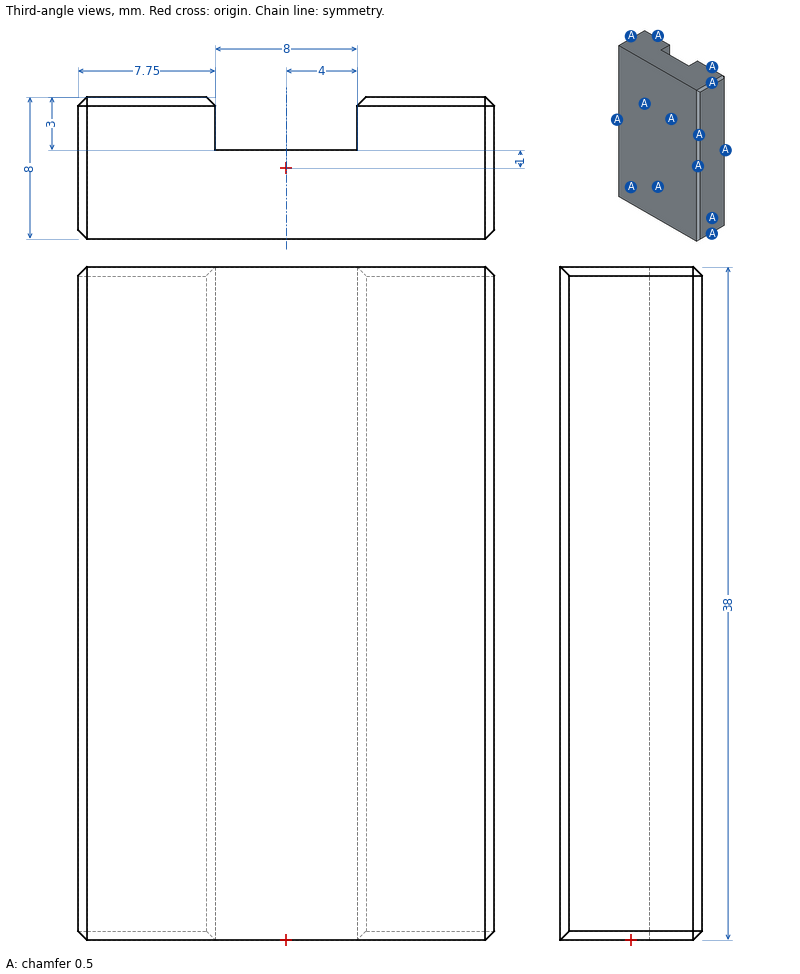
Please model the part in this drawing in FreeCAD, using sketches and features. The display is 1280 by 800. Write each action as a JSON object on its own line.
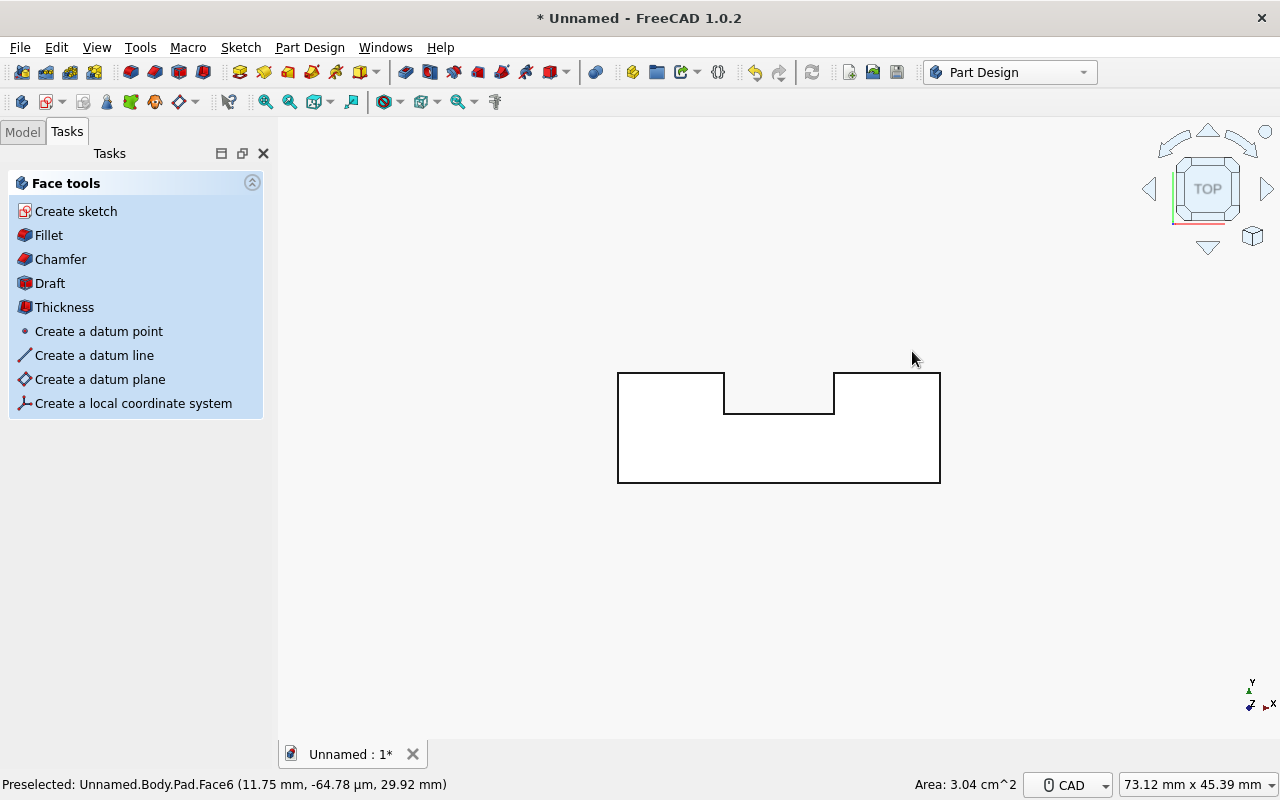
{"action": "key", "text": "1"}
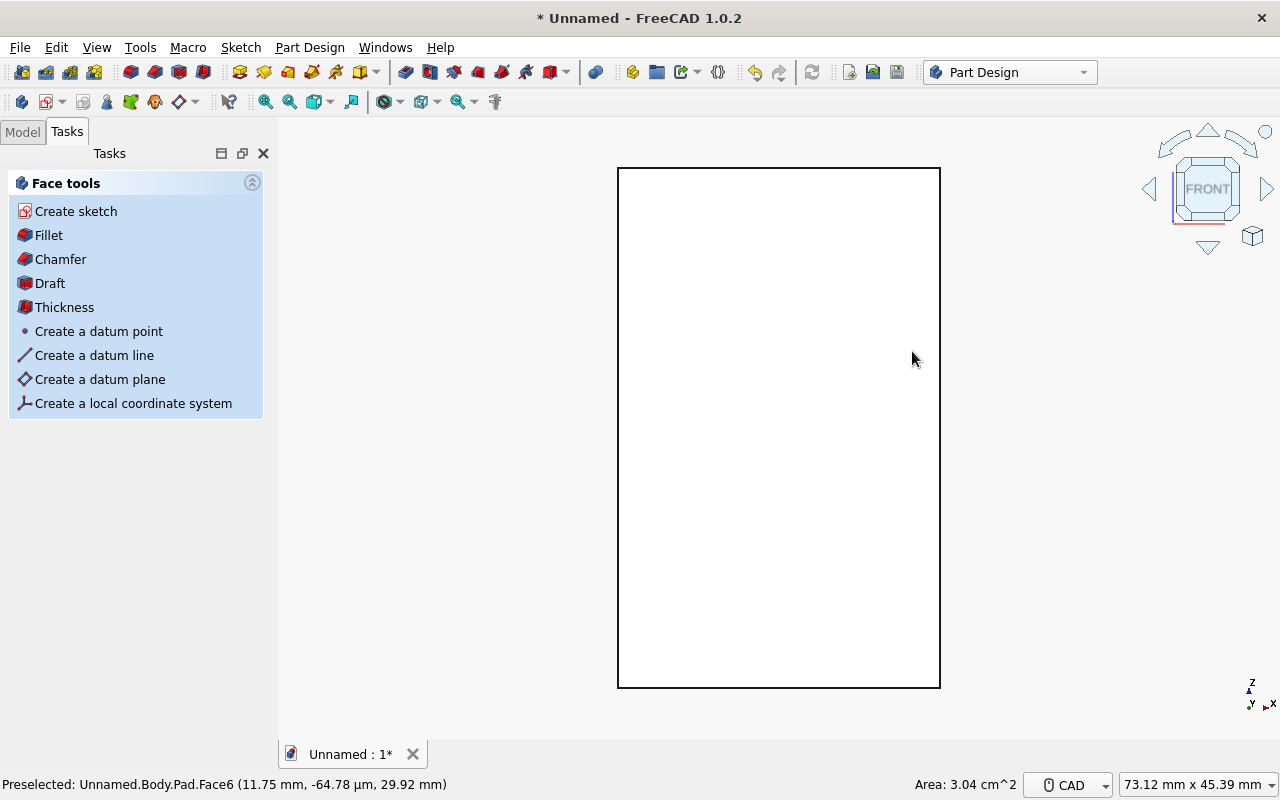
{"action": "key", "text": "3"}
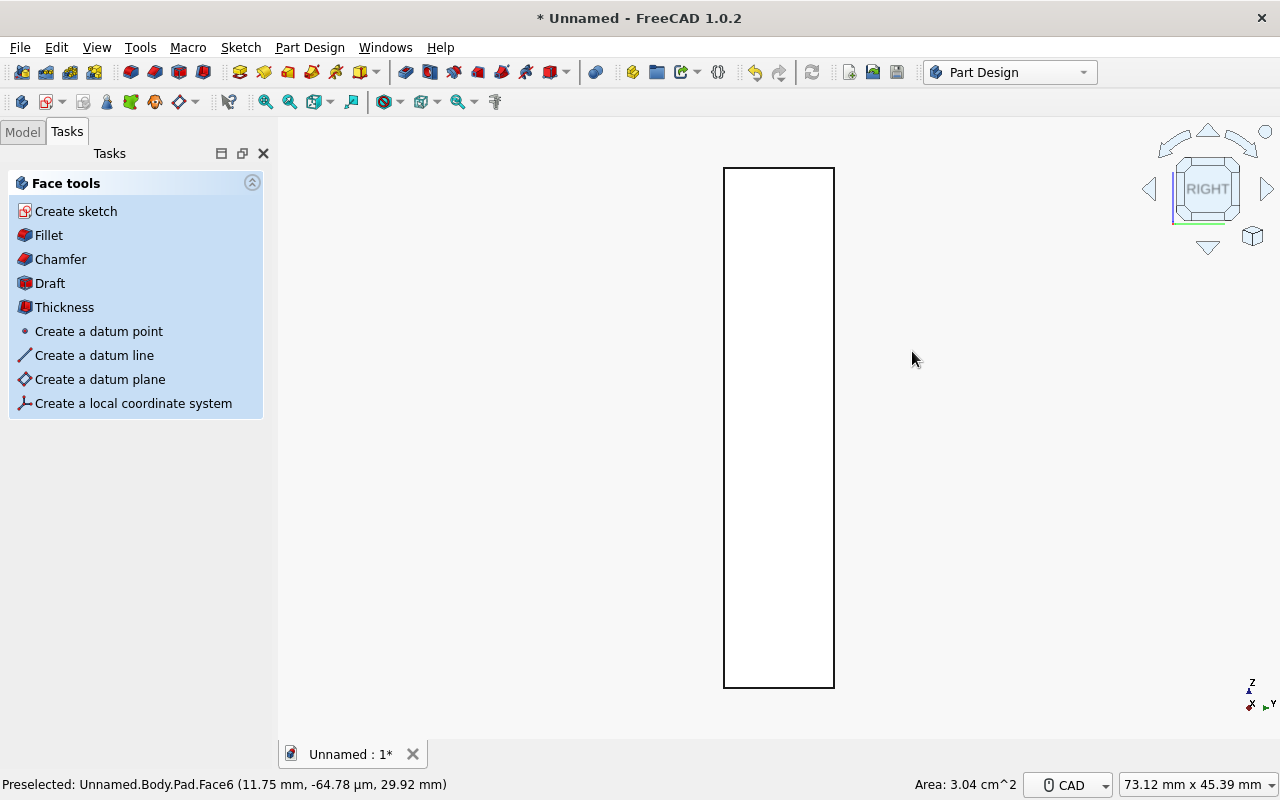
{"action": "key", "text": "5"}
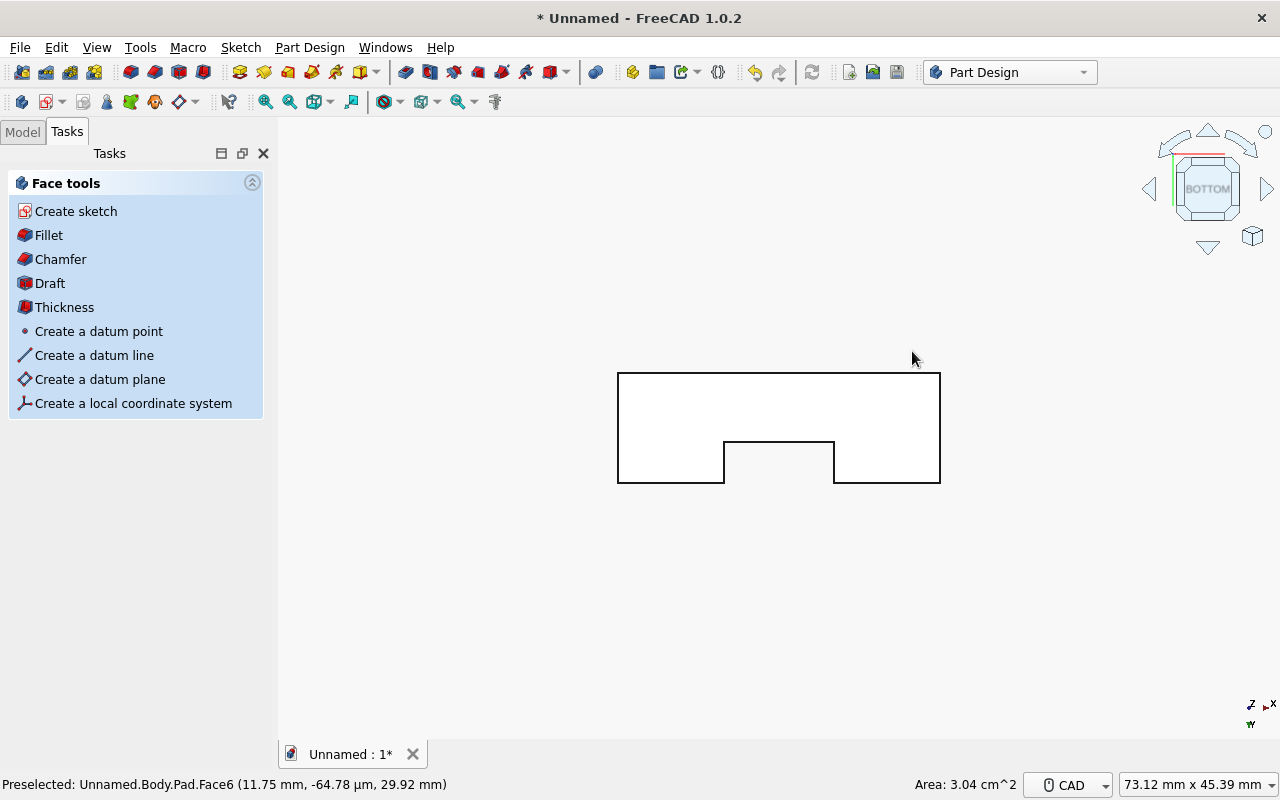
{"action": "left_click", "coordinate": [266, 102]}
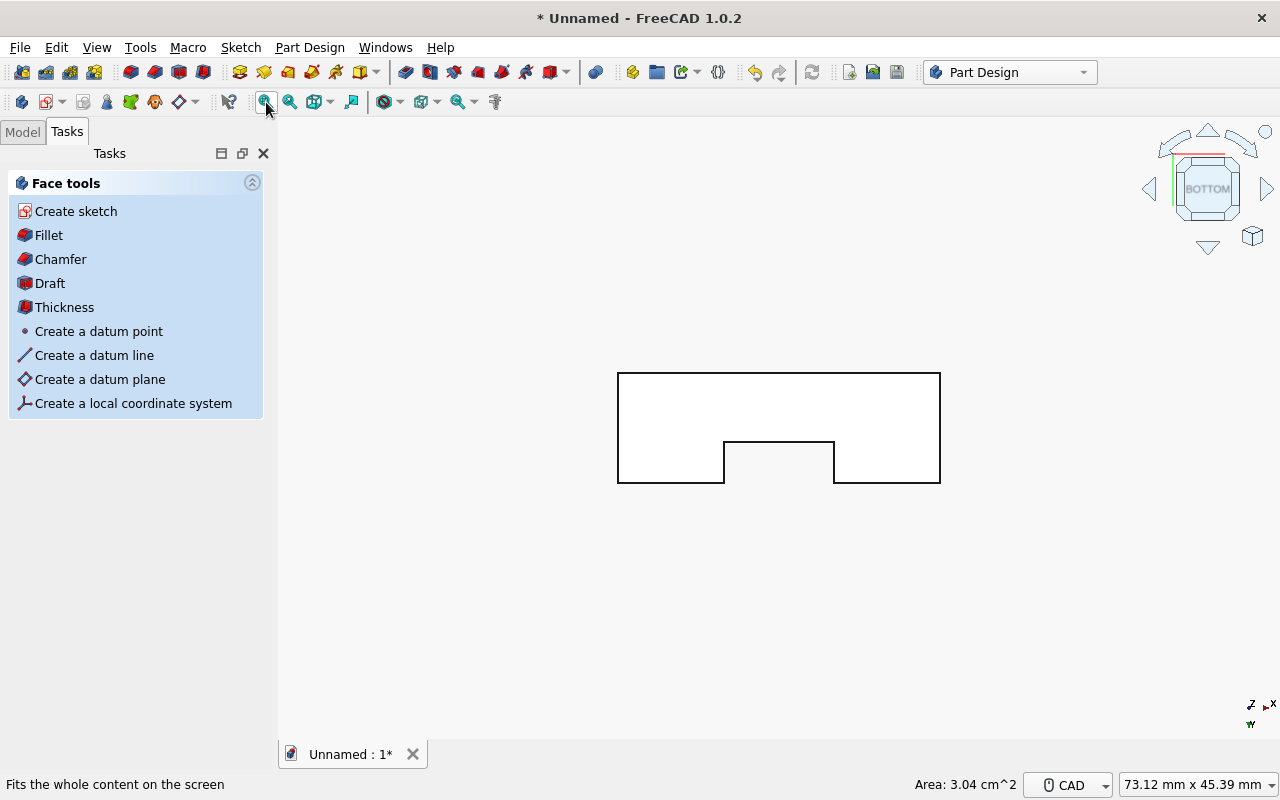
{"action": "key", "text": "4"}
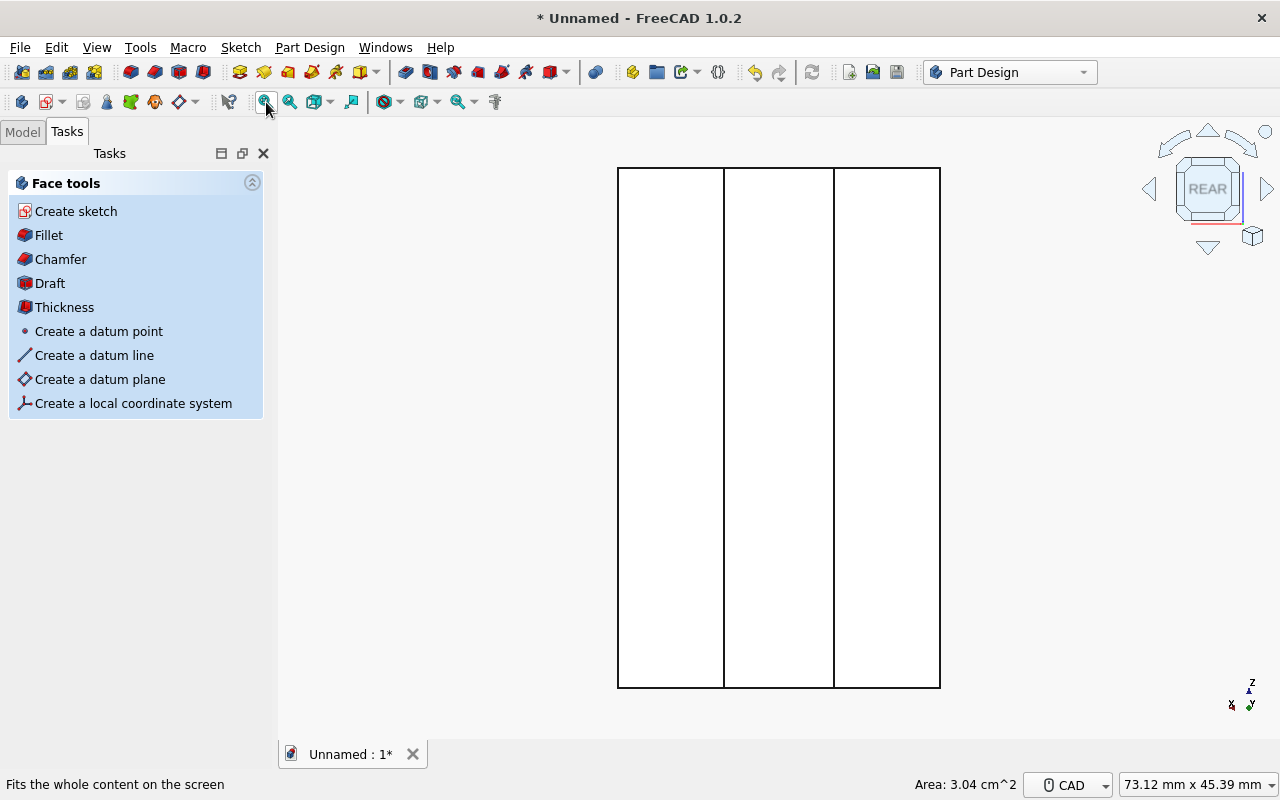
{"action": "left_click", "coordinate": [887, 278], "text": "ctrl"}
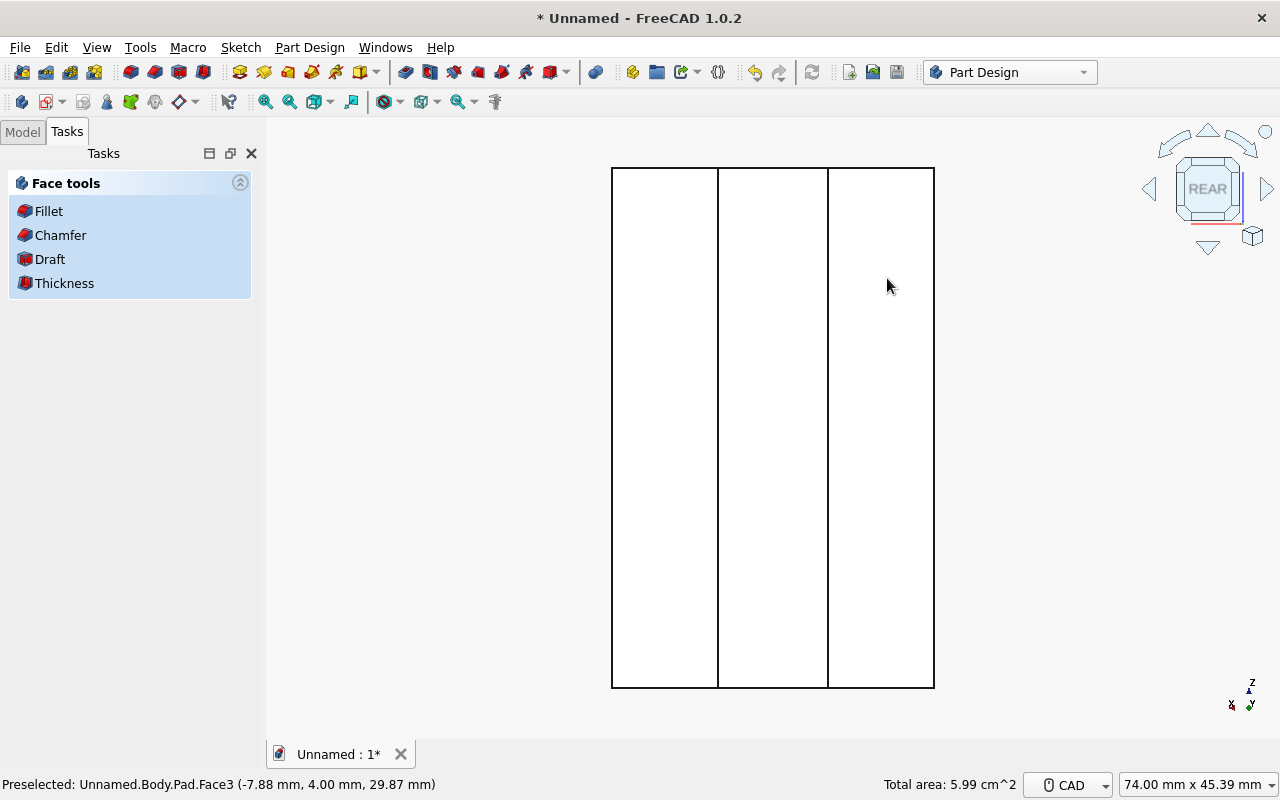
{"action": "left_click", "coordinate": [665, 278], "text": "ctrl"}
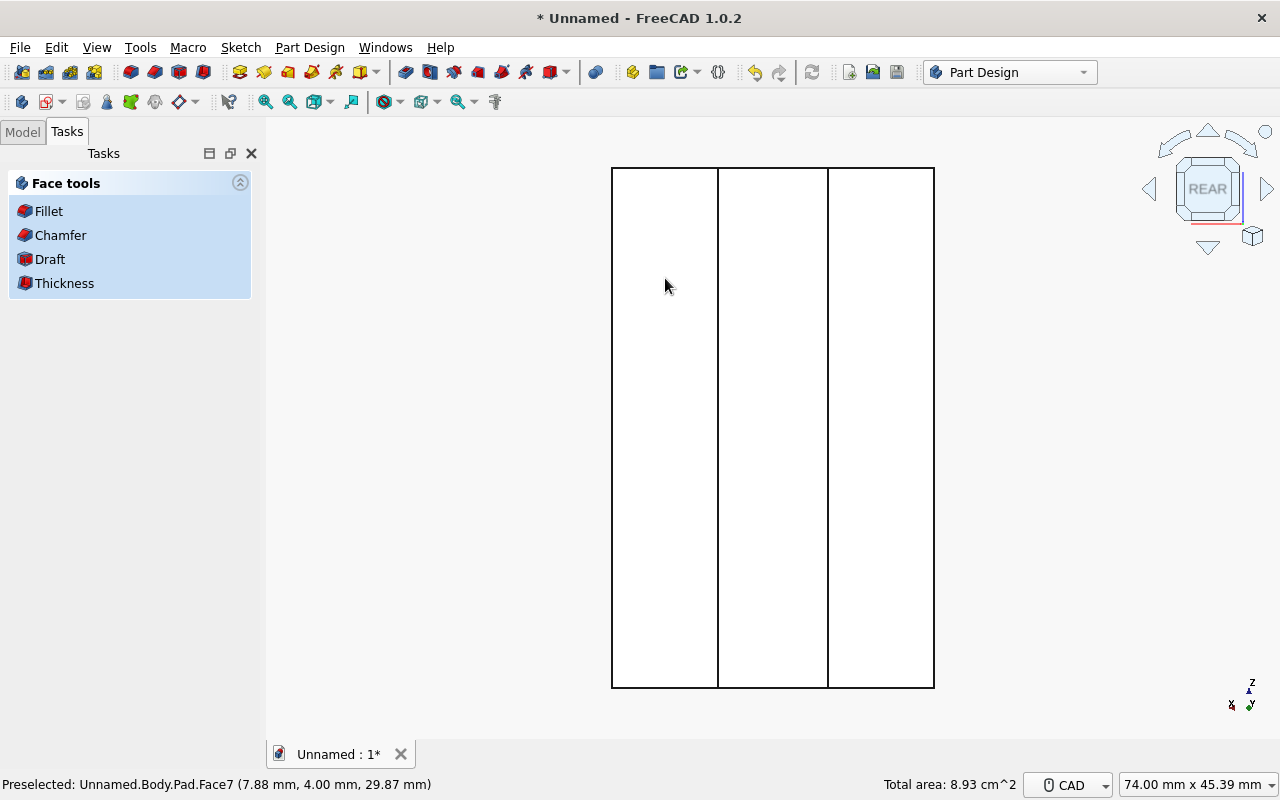
{"action": "key", "text": "6"}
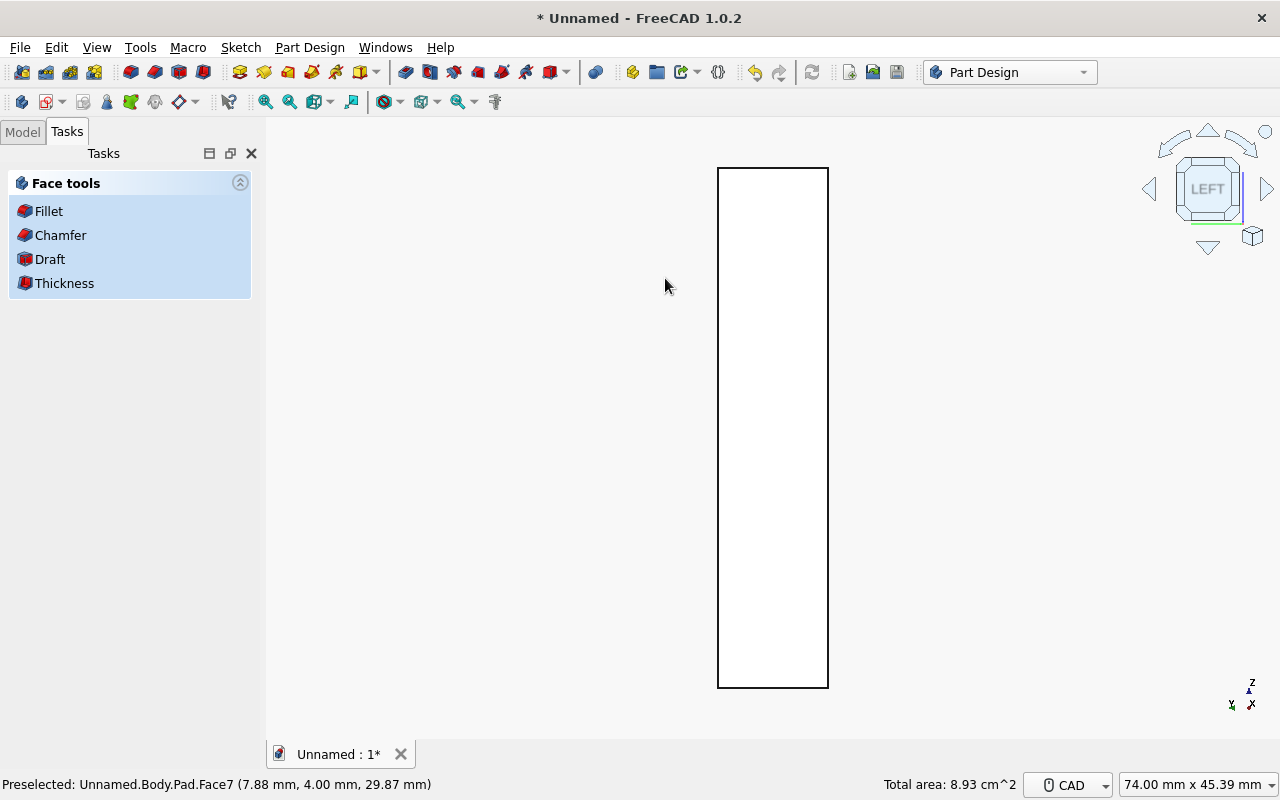
{"action": "left_click", "coordinate": [773, 278], "text": "ctrl"}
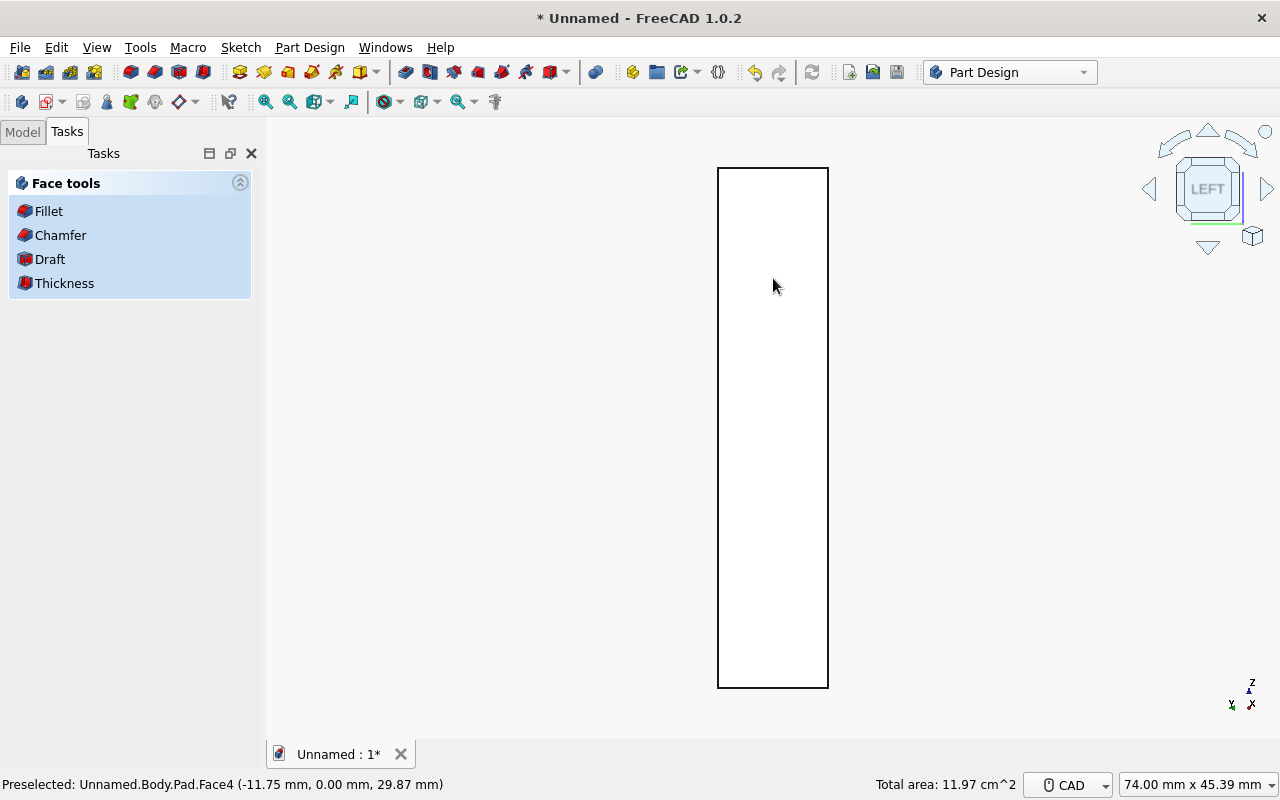
{"action": "left_click", "coordinate": [156, 72]}